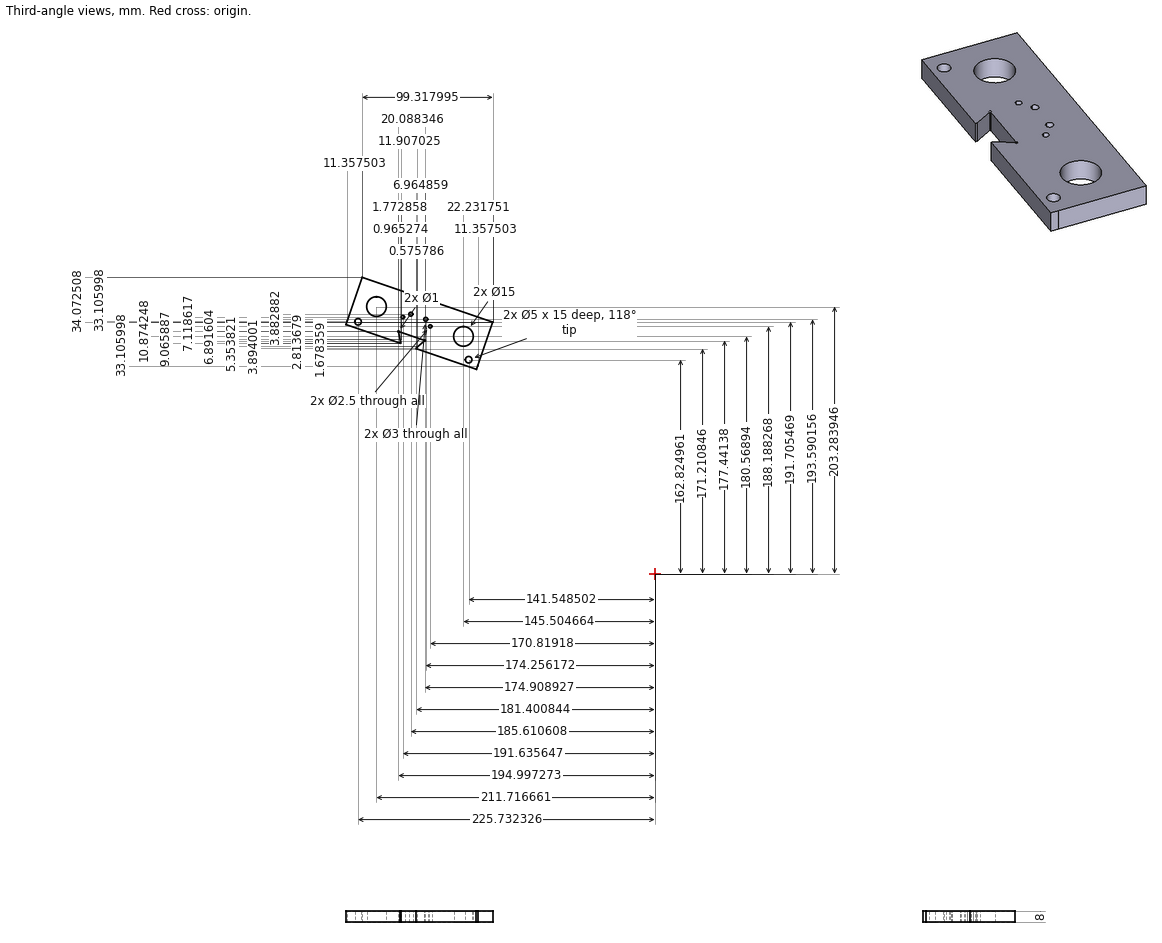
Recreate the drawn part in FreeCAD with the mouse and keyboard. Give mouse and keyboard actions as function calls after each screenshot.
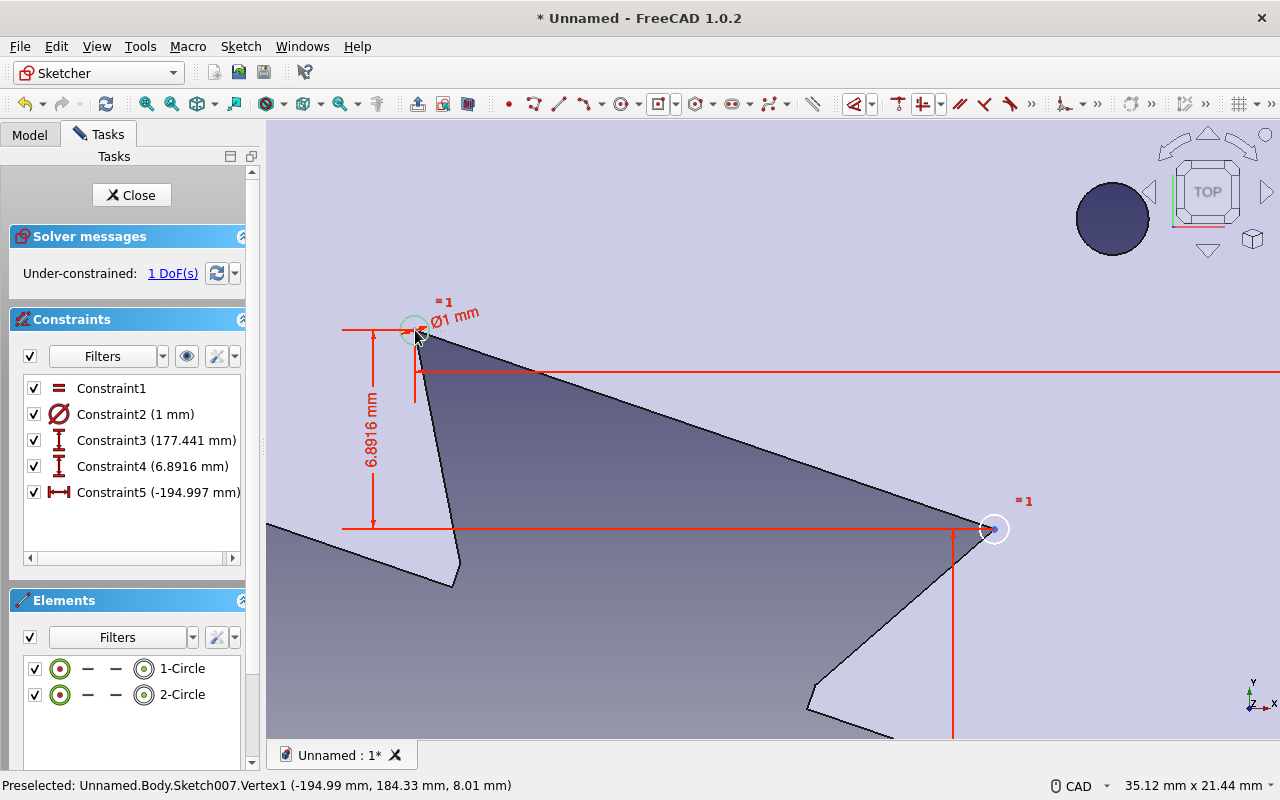
click(994, 529)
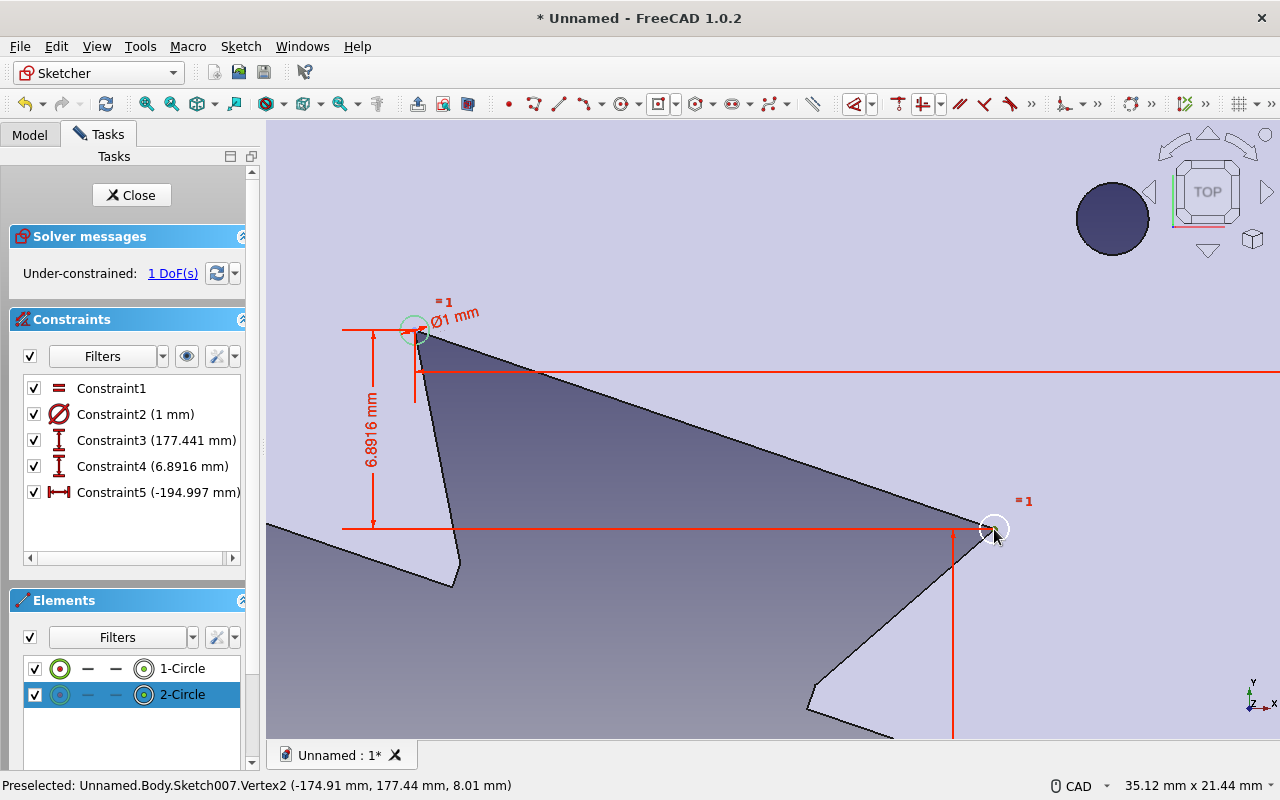
click(872, 104)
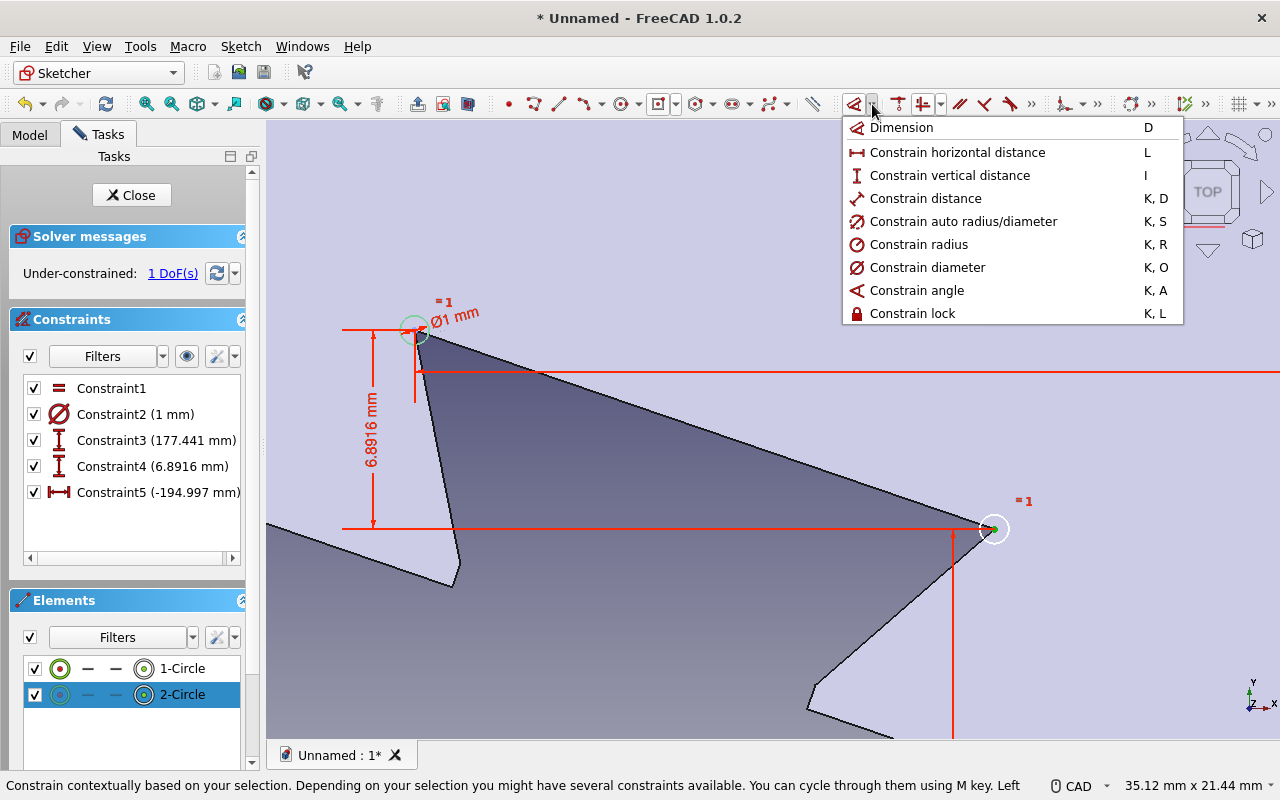
click(1013, 152)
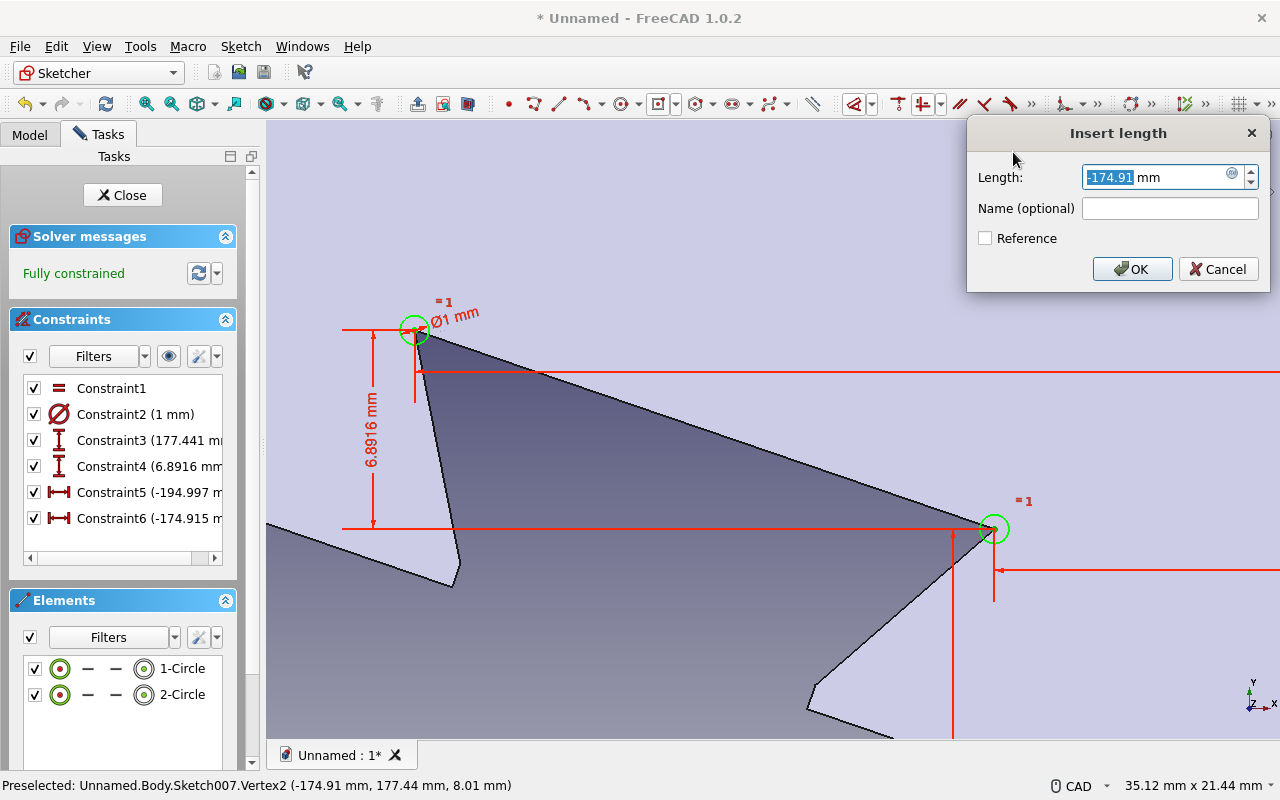
text(-174.908927)
key(Return)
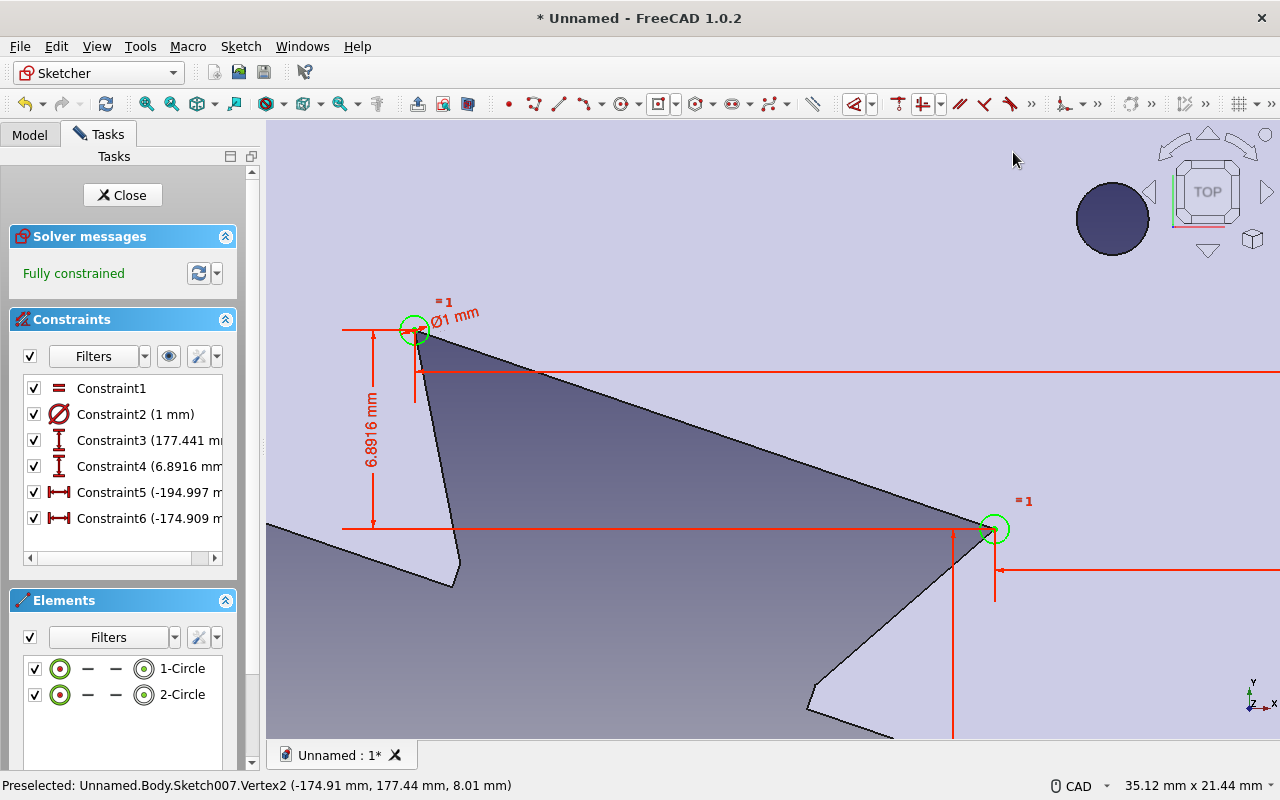
click(123, 195)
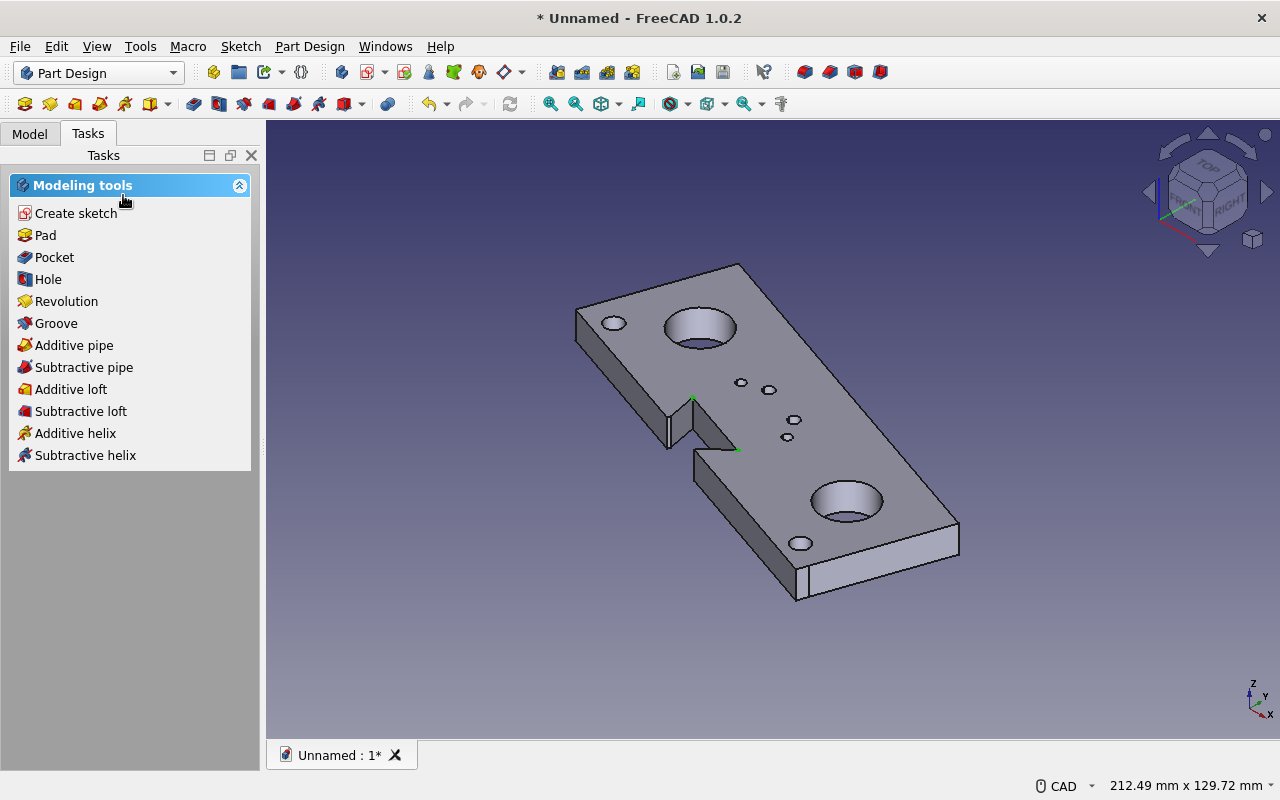
click(194, 104)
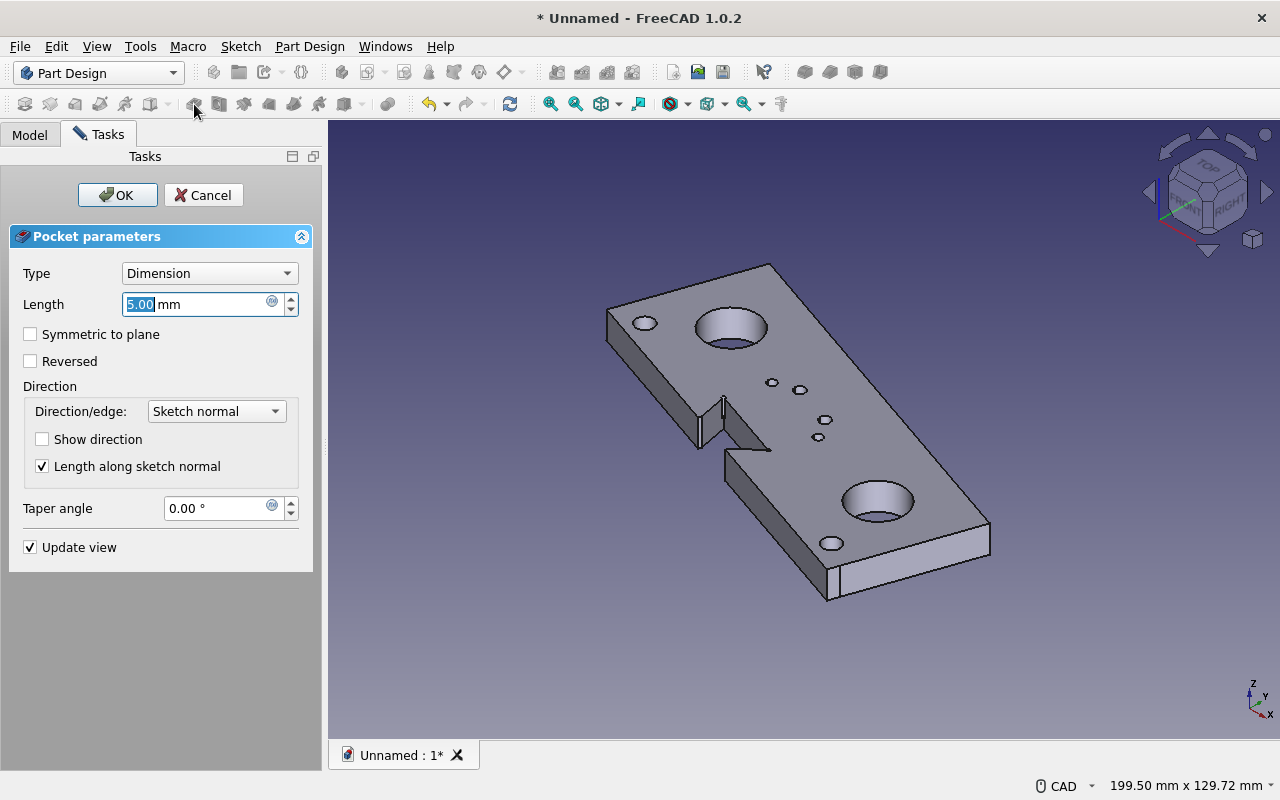
click(210, 274)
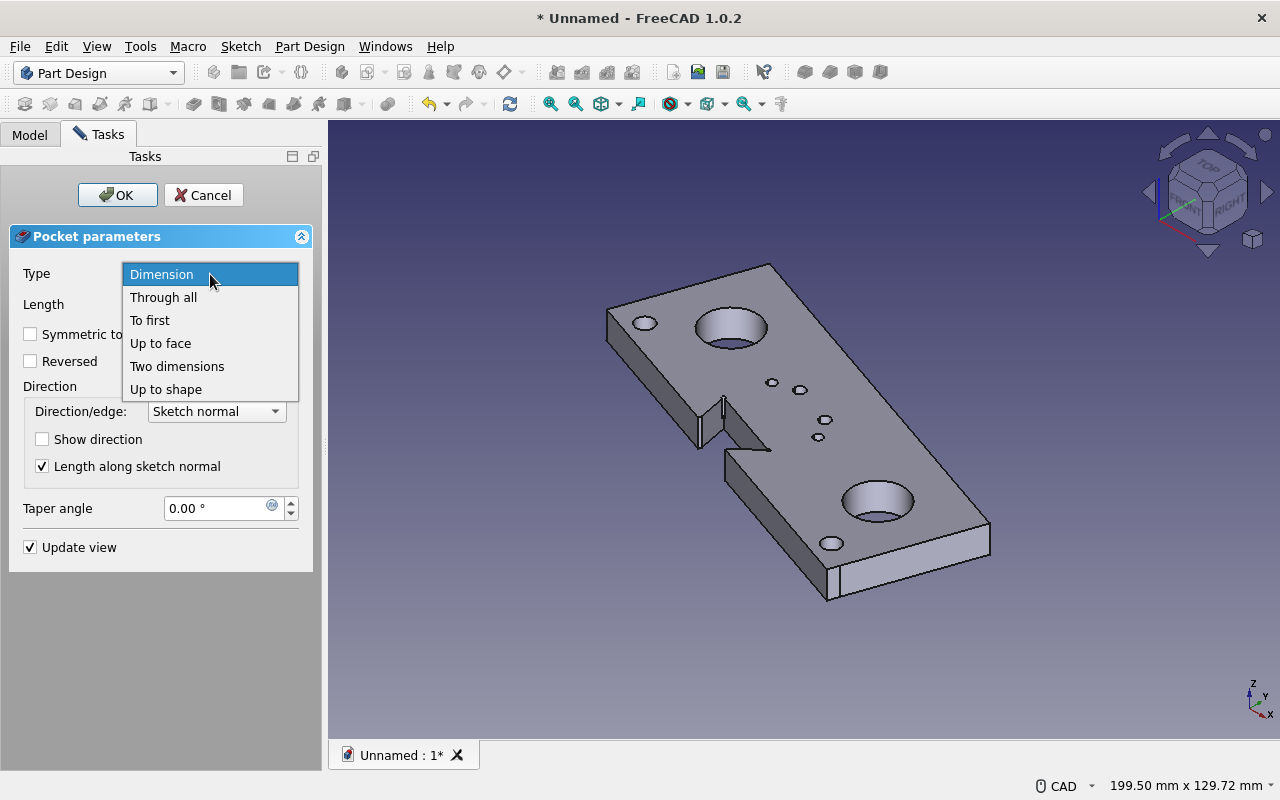
click(208, 298)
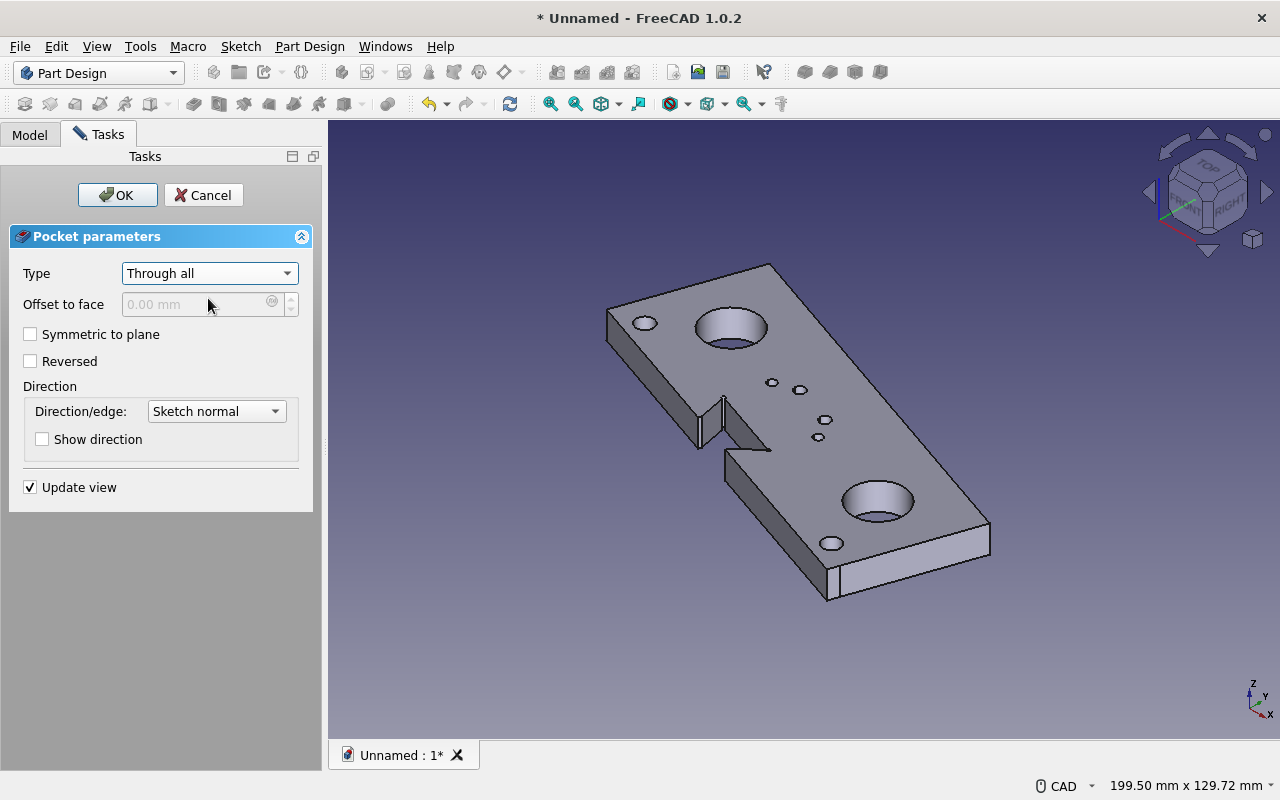
click(118, 195)